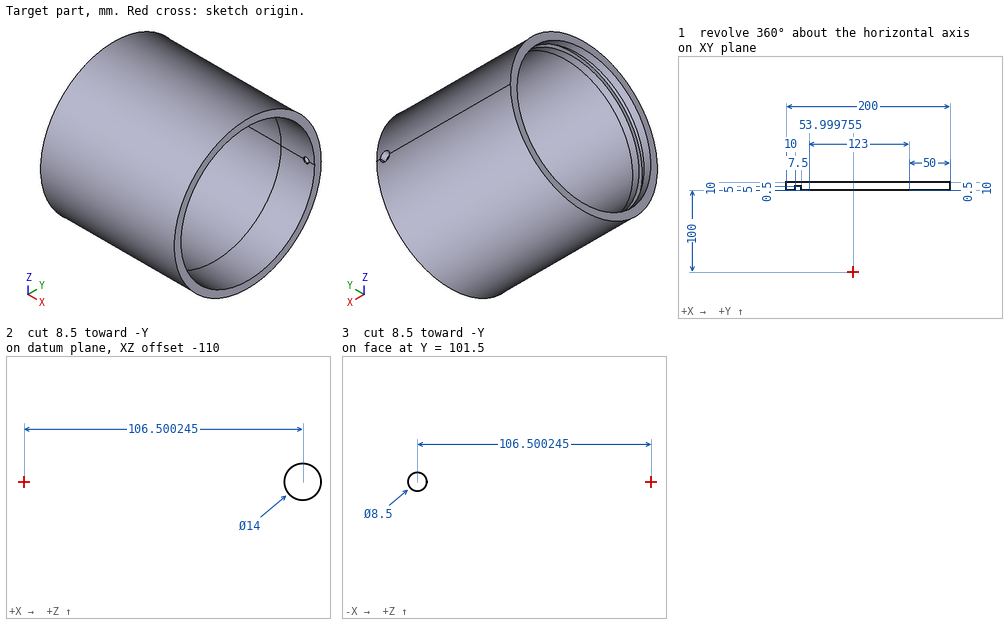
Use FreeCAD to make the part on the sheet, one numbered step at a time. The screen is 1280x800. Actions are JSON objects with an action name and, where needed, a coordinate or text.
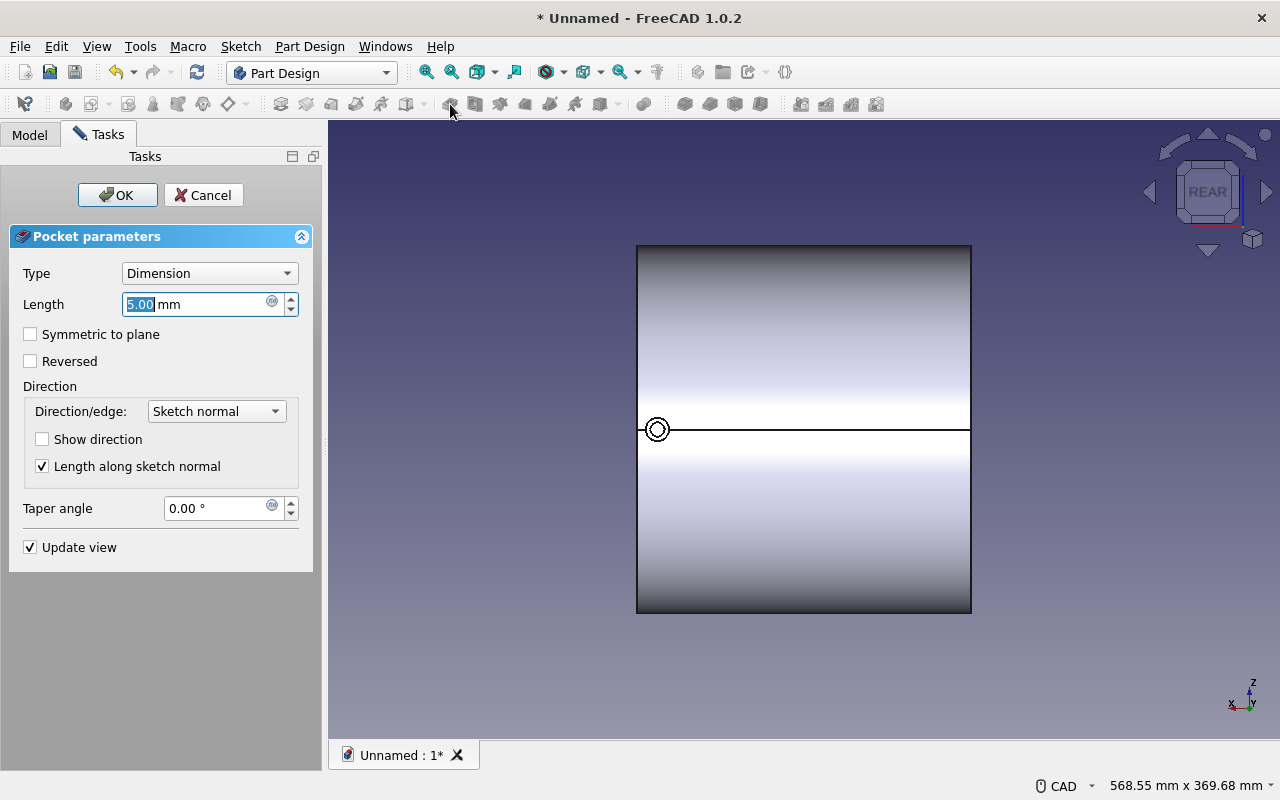
{"action": "type", "text": "8.5"}
{"action": "key", "text": "Tab"}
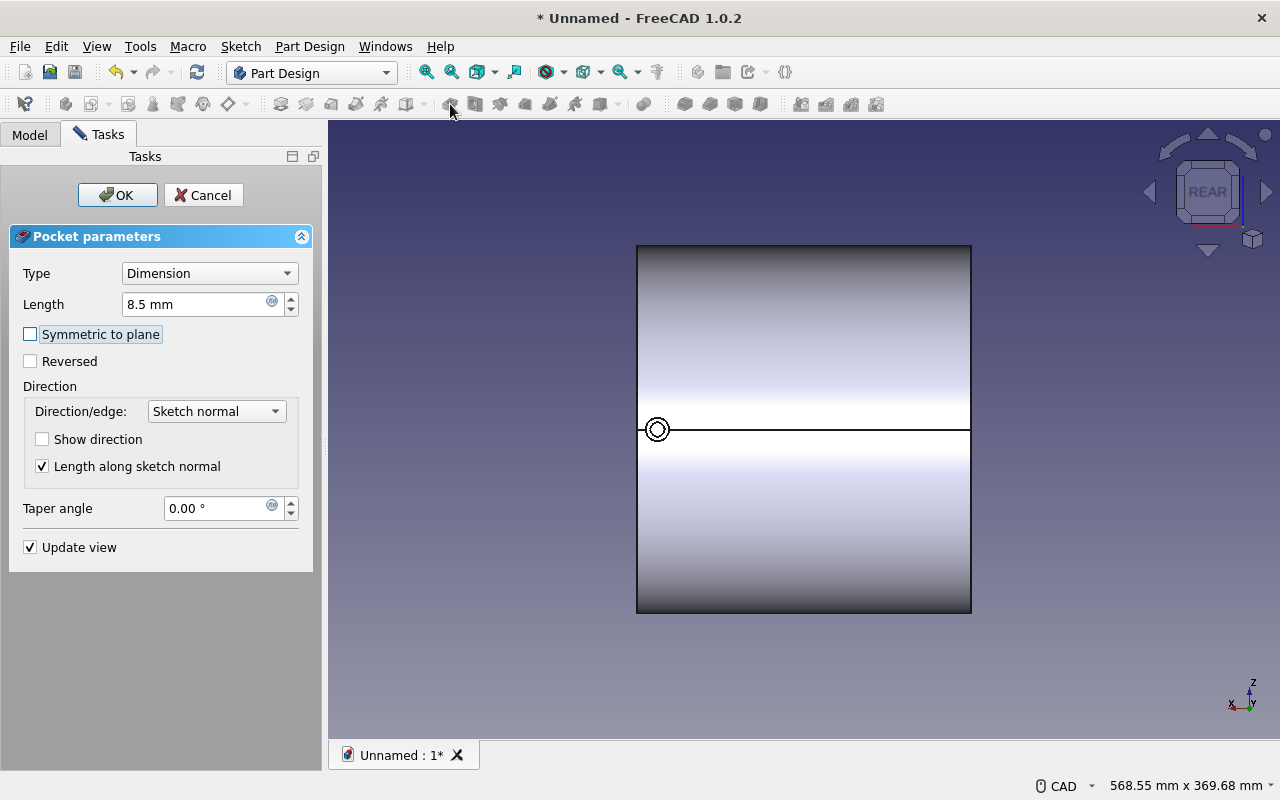
{"action": "left_click", "coordinate": [118, 195]}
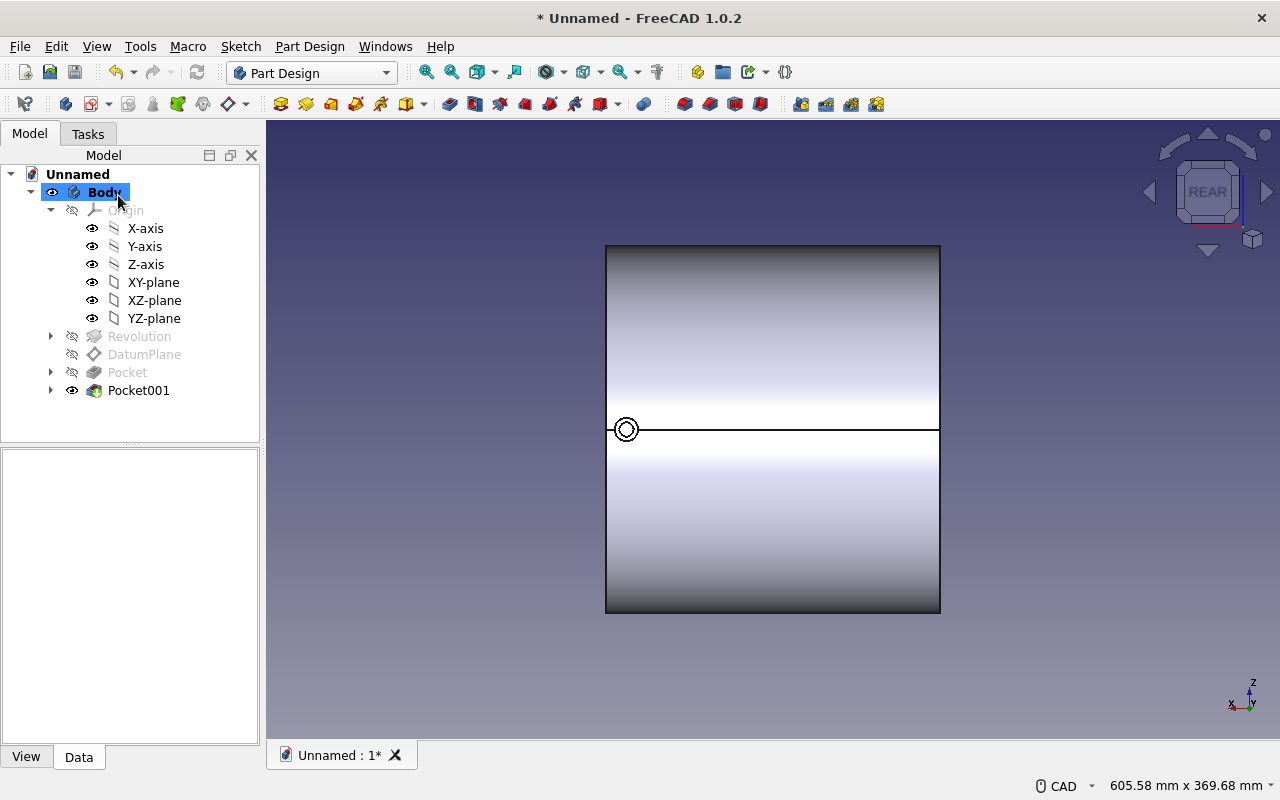
{"action": "key", "text": "0"}